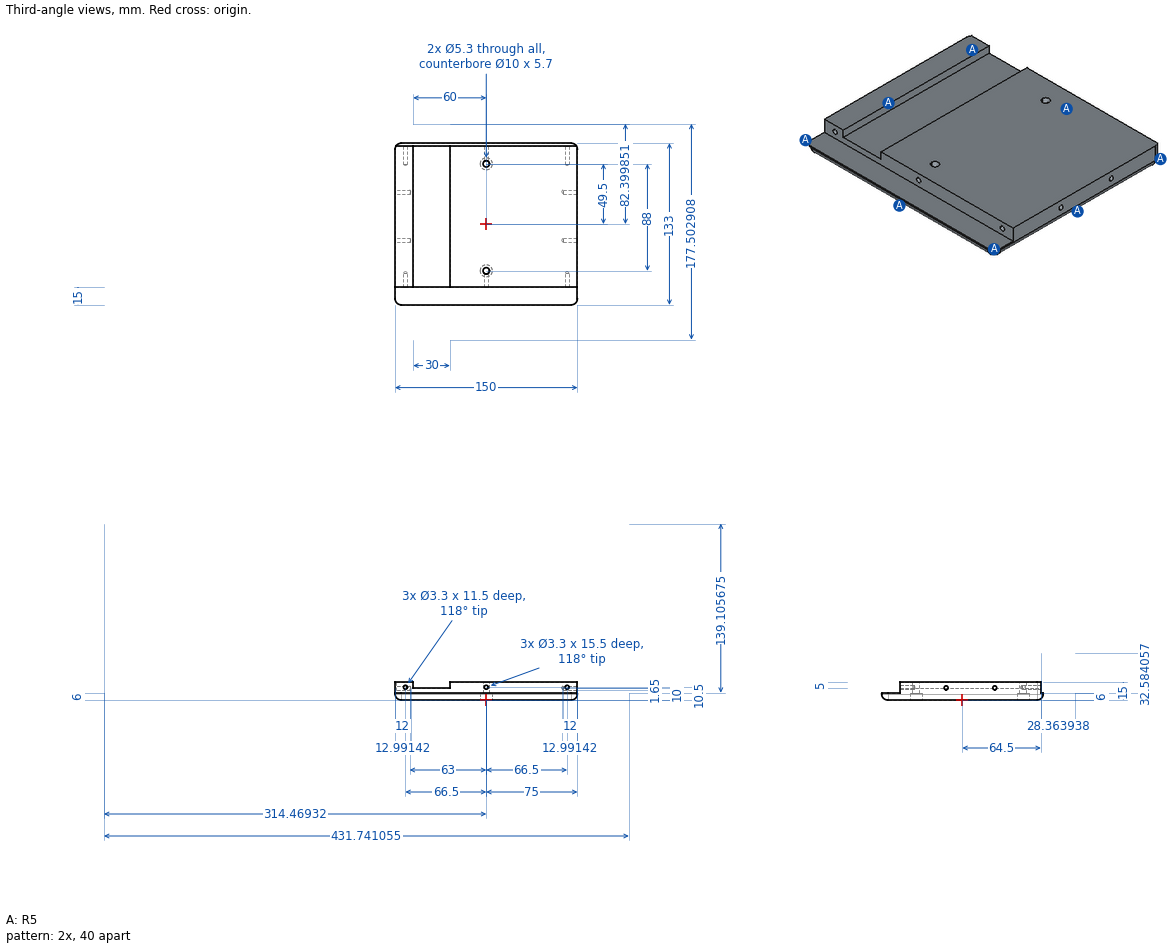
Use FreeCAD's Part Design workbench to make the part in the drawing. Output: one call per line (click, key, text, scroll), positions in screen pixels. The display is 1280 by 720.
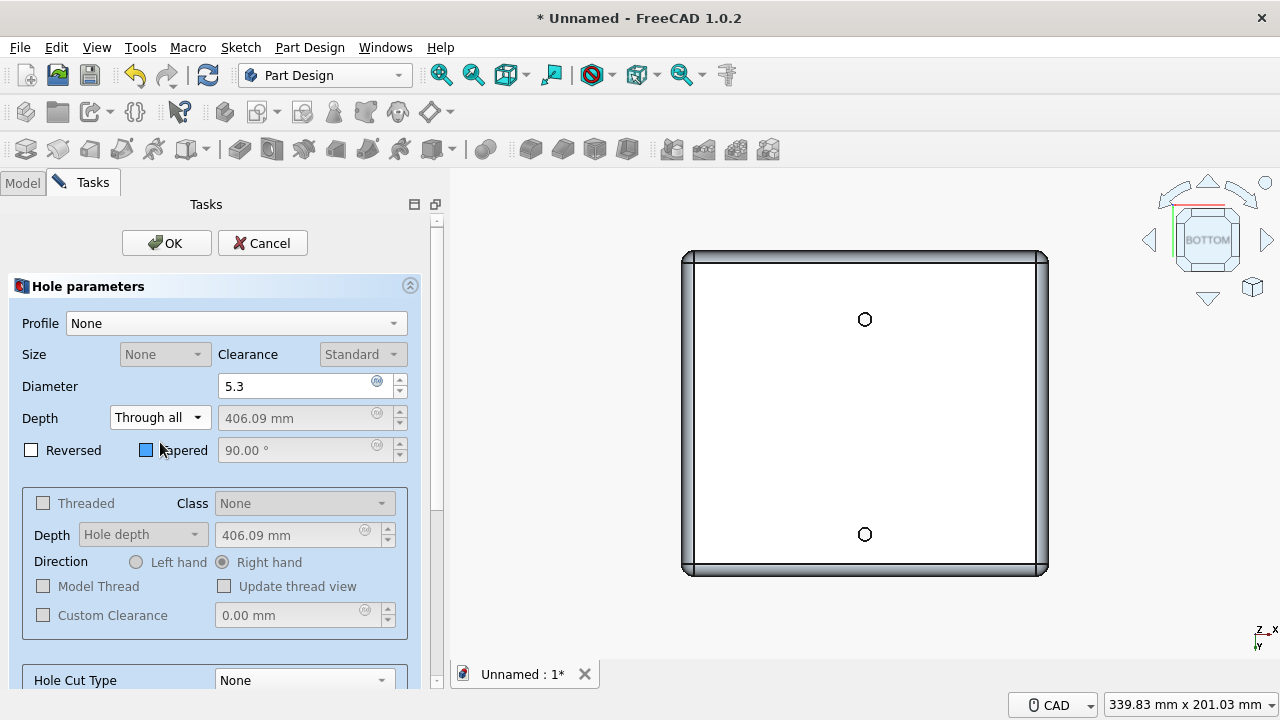
scroll(437, 451, down, 2)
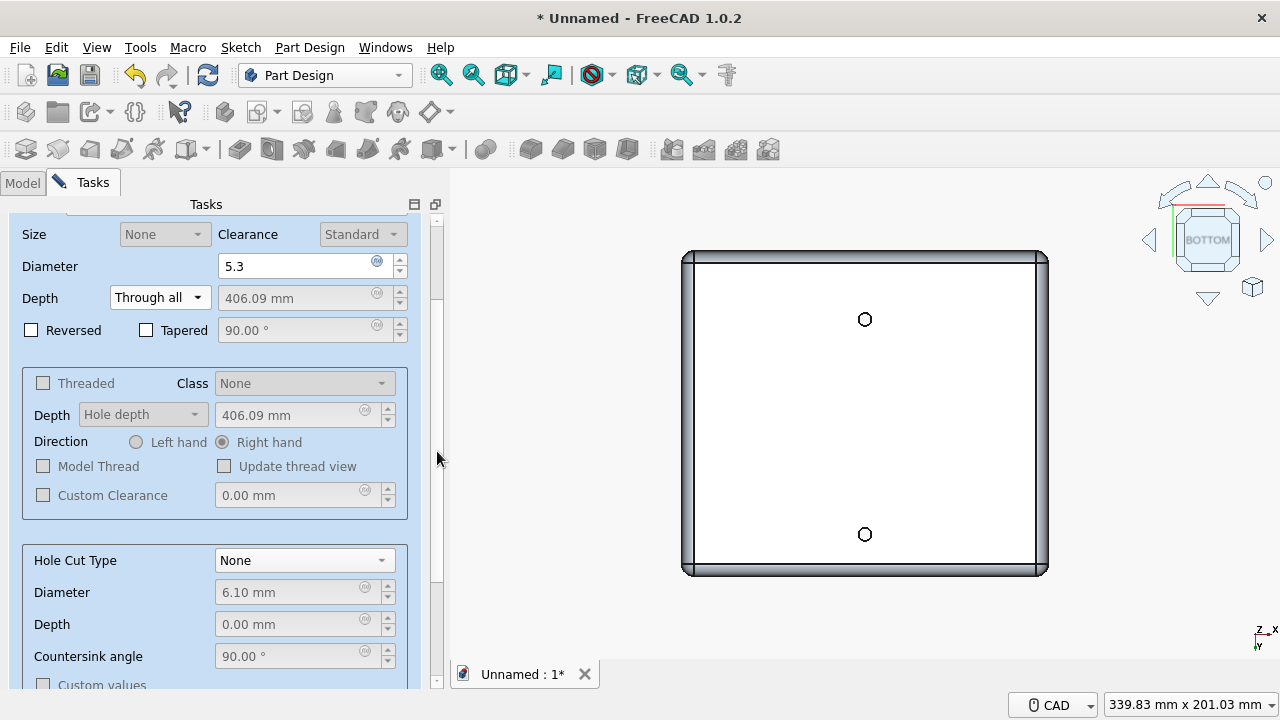
click(306, 560)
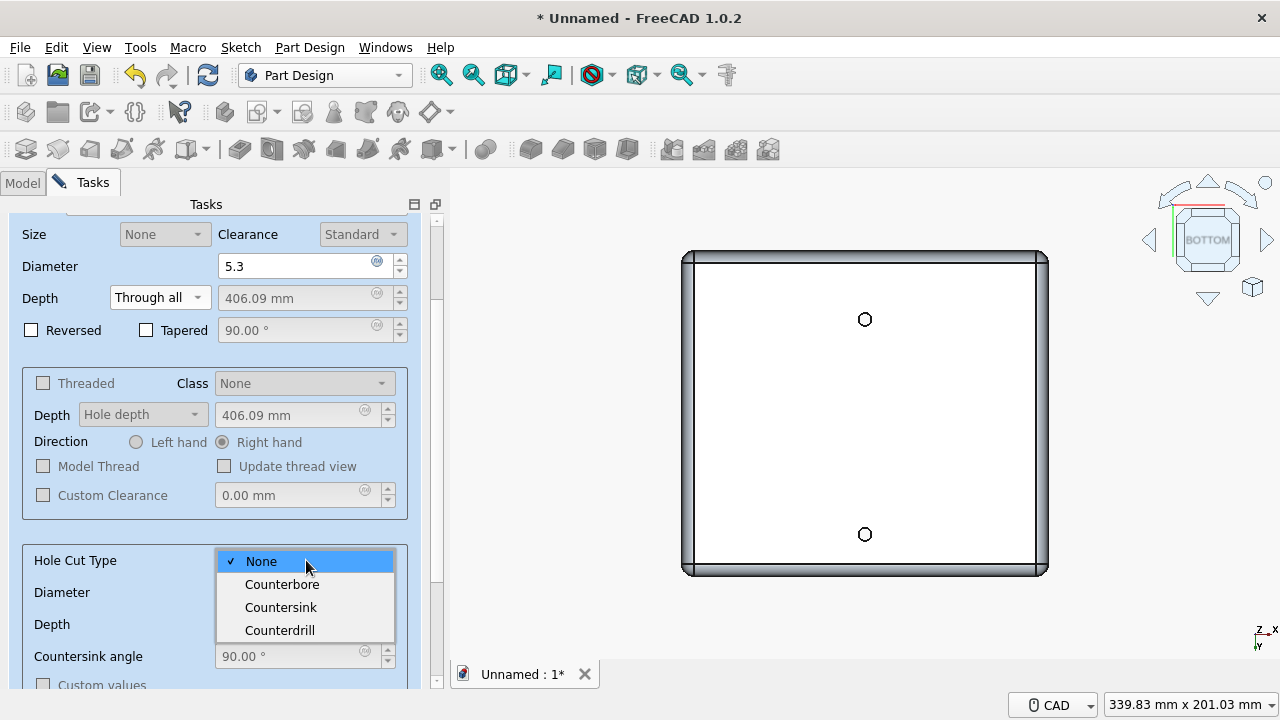
click(304, 584)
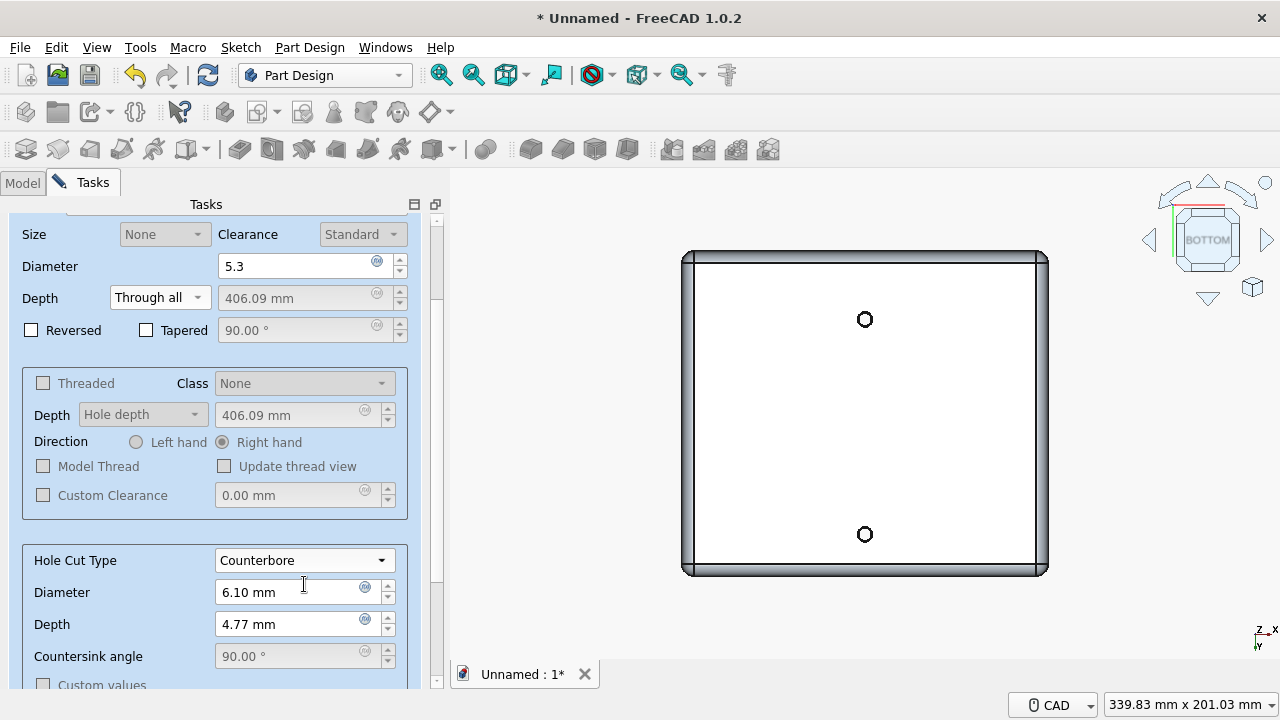
triple_click(298, 592)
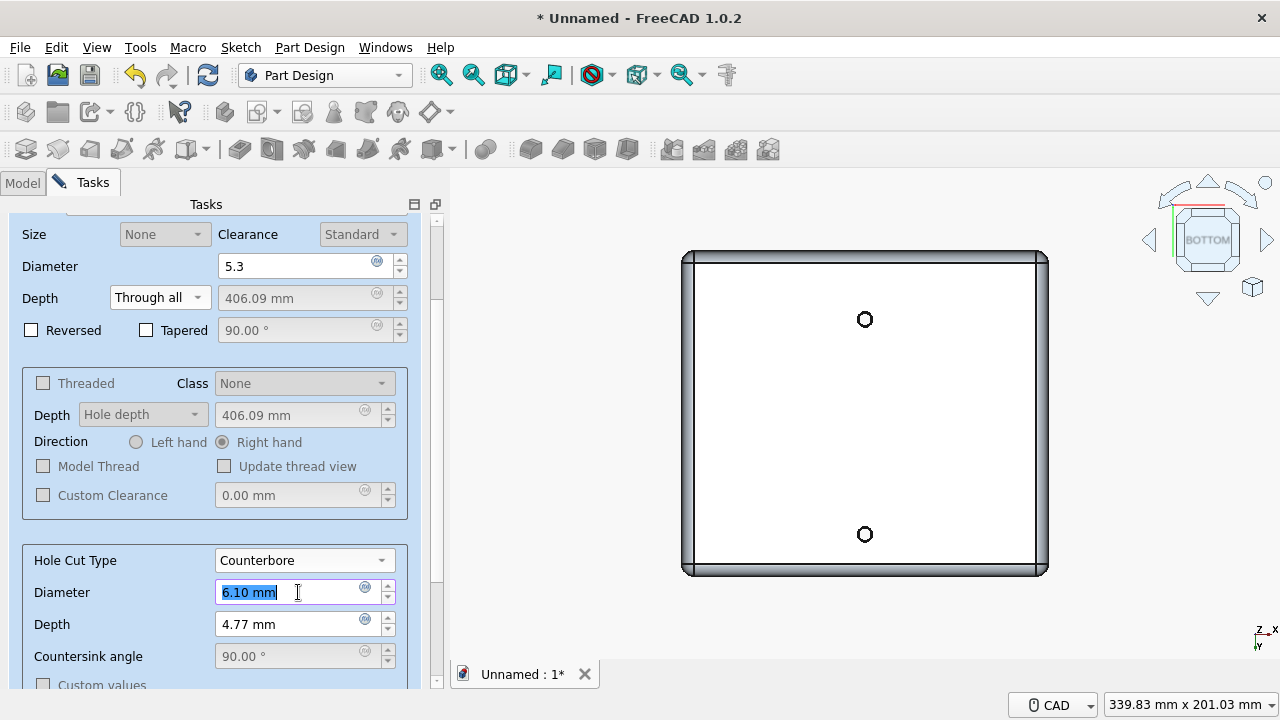
text(10)
key(Tab)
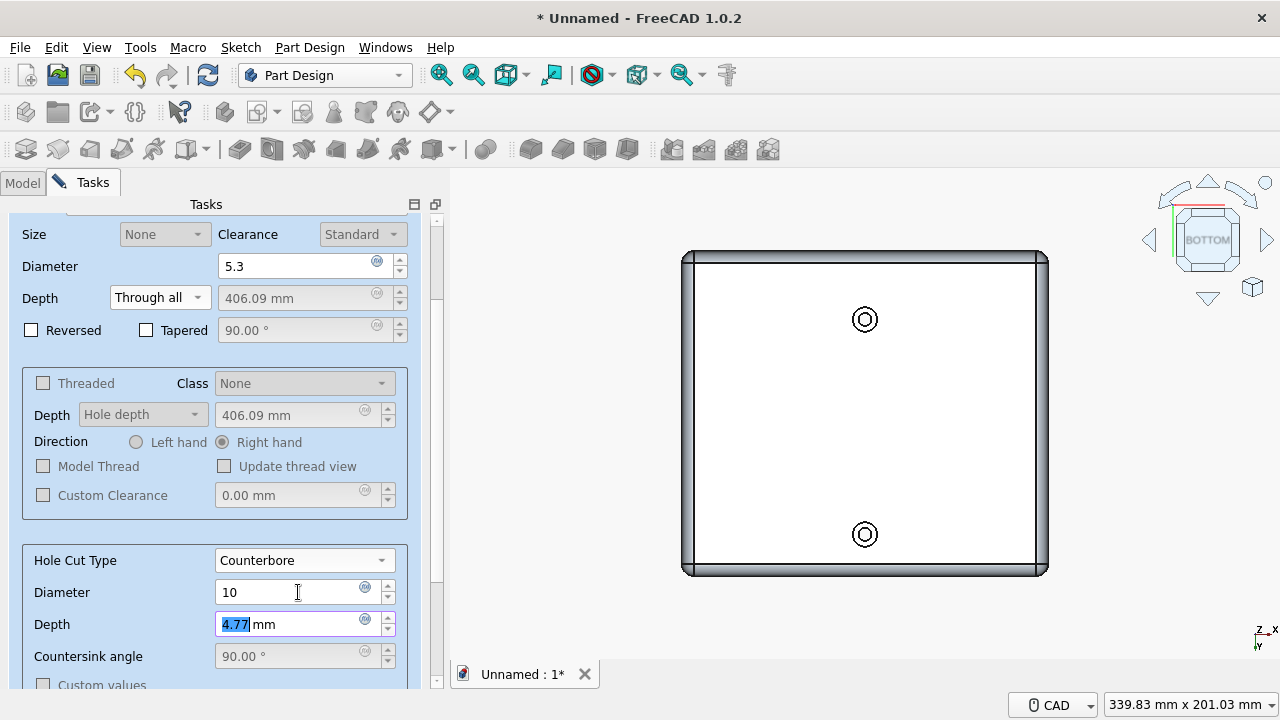
text(5.7)
key(Tab)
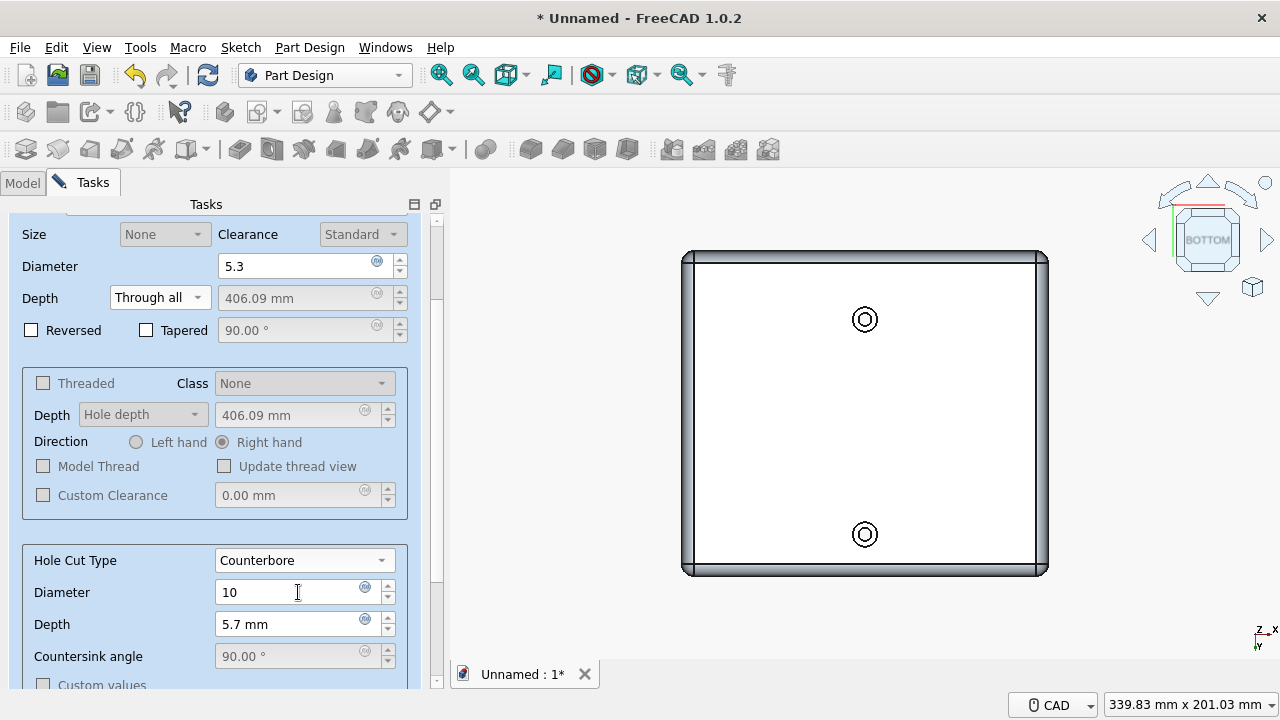
scroll(437, 451, up, 3)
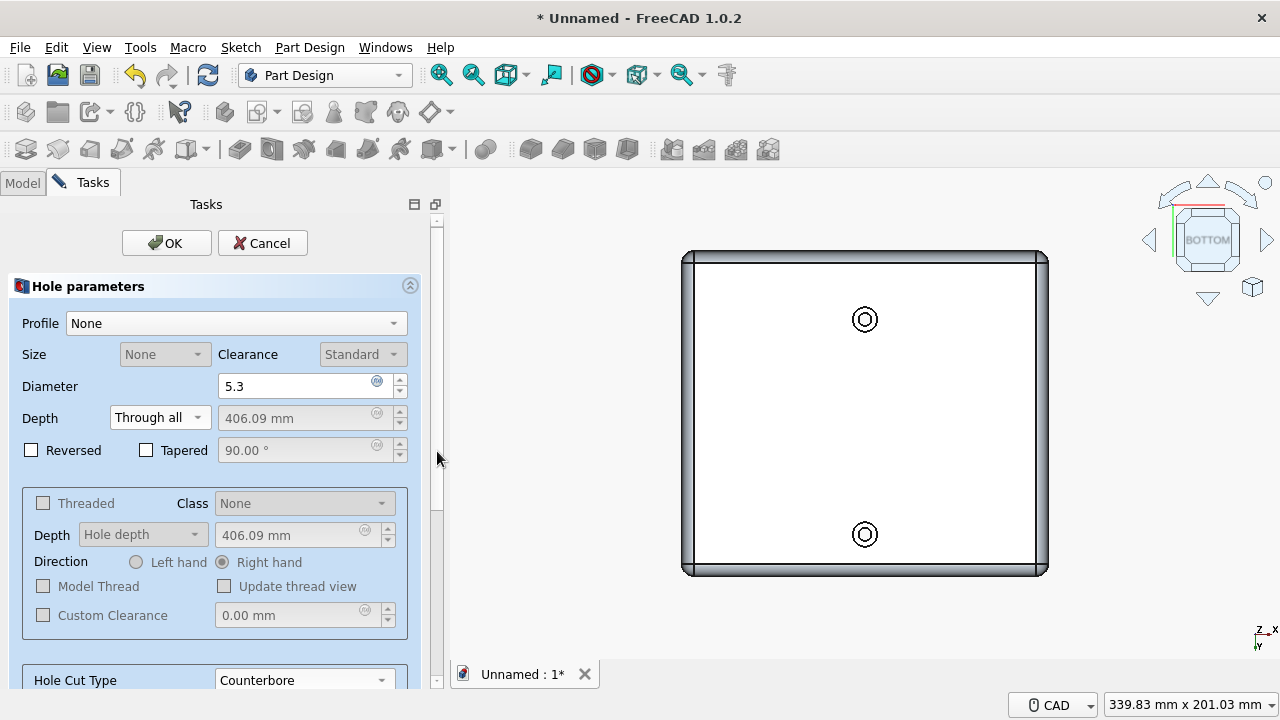
click(167, 243)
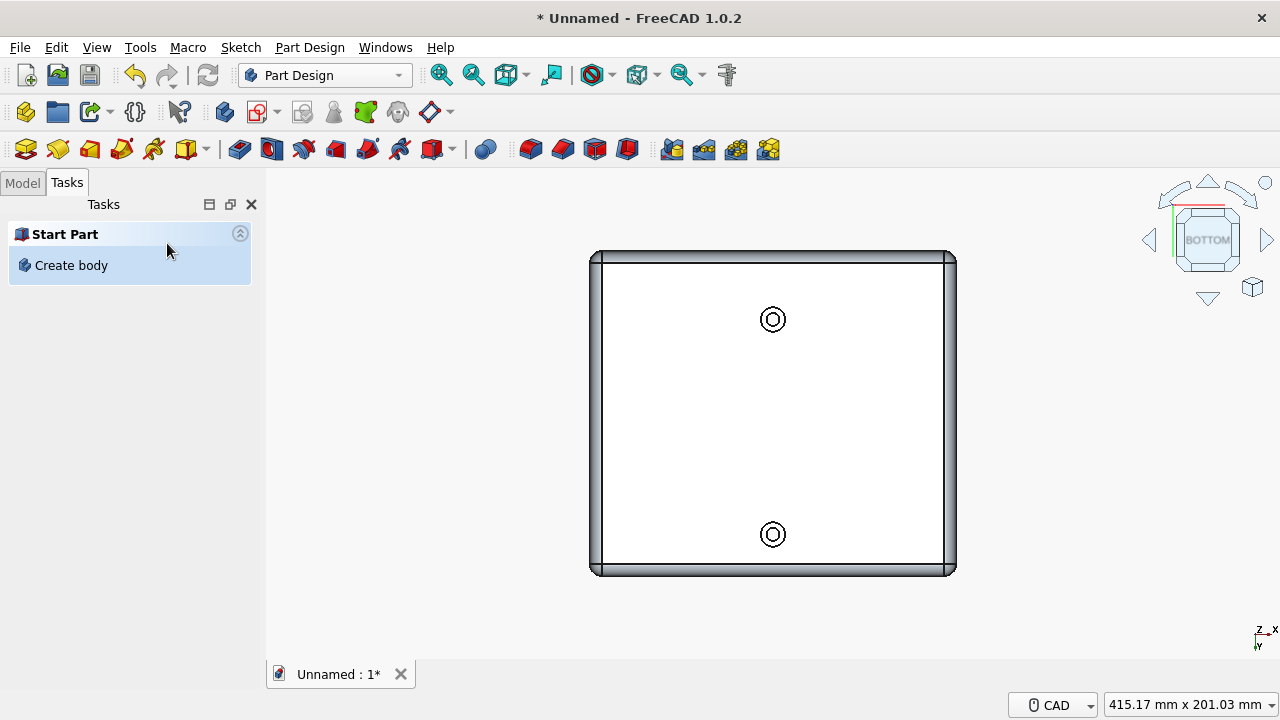
key(4)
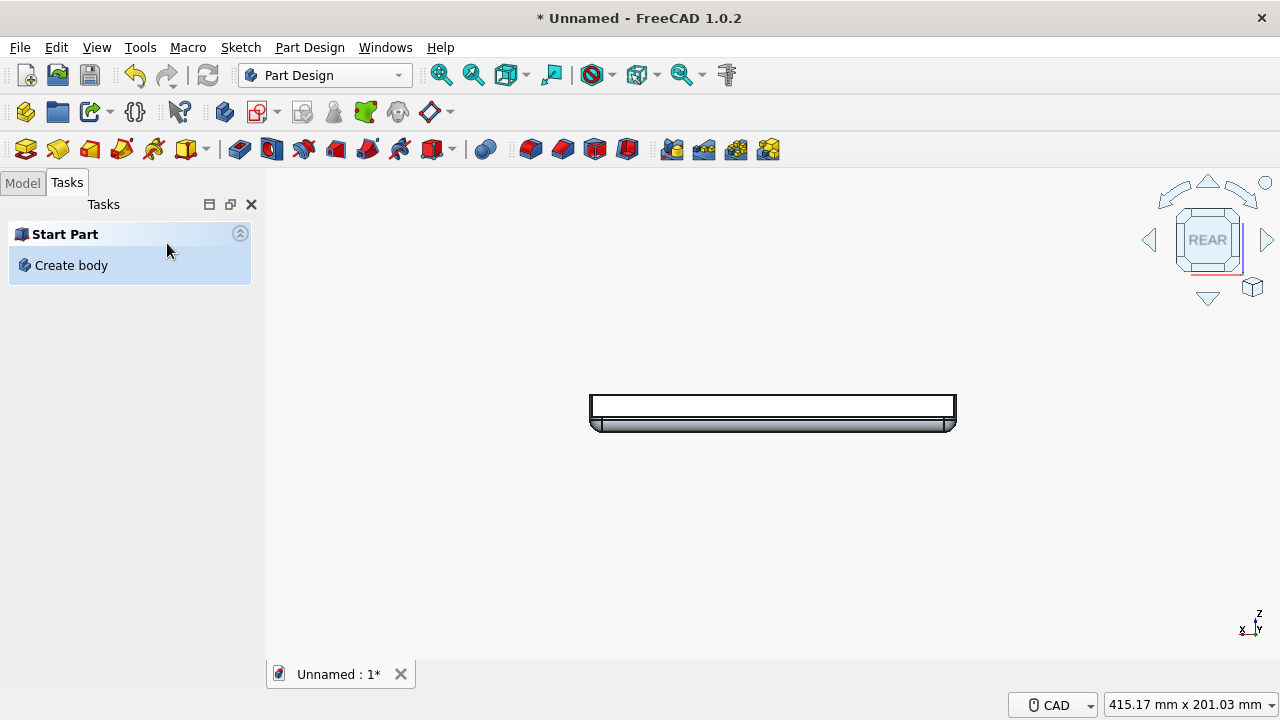
click(442, 76)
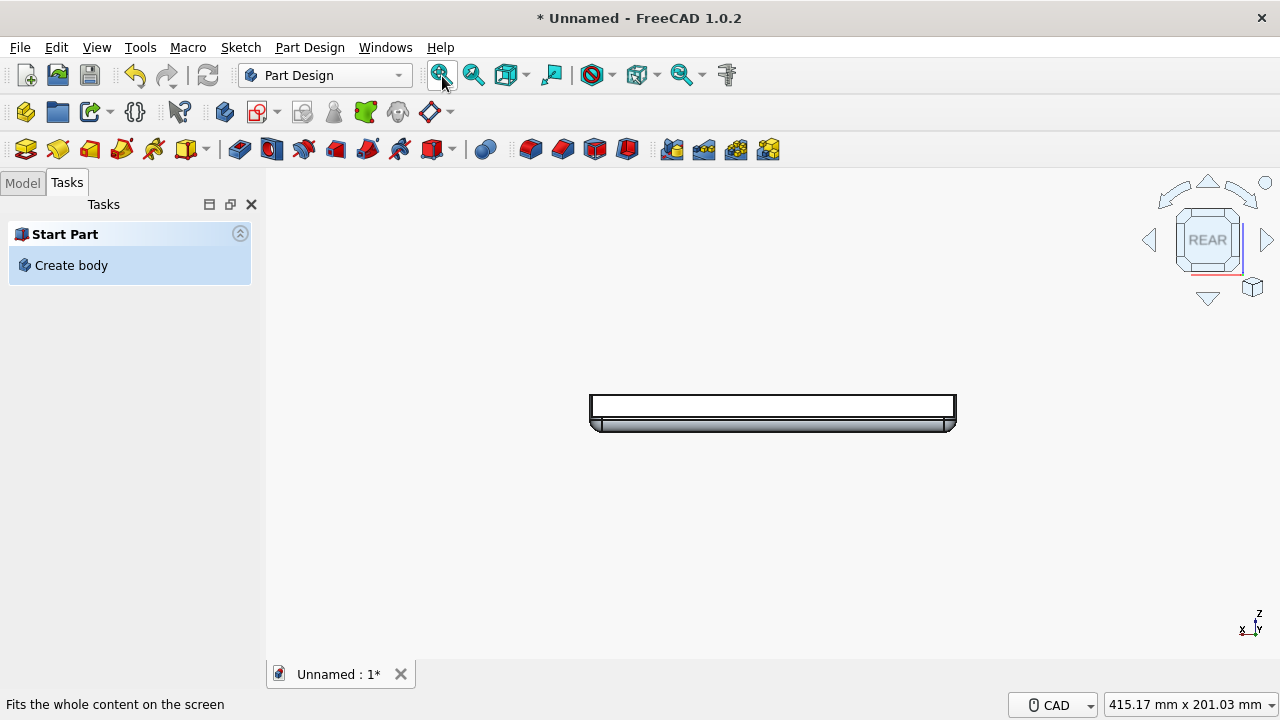
click(618, 405)